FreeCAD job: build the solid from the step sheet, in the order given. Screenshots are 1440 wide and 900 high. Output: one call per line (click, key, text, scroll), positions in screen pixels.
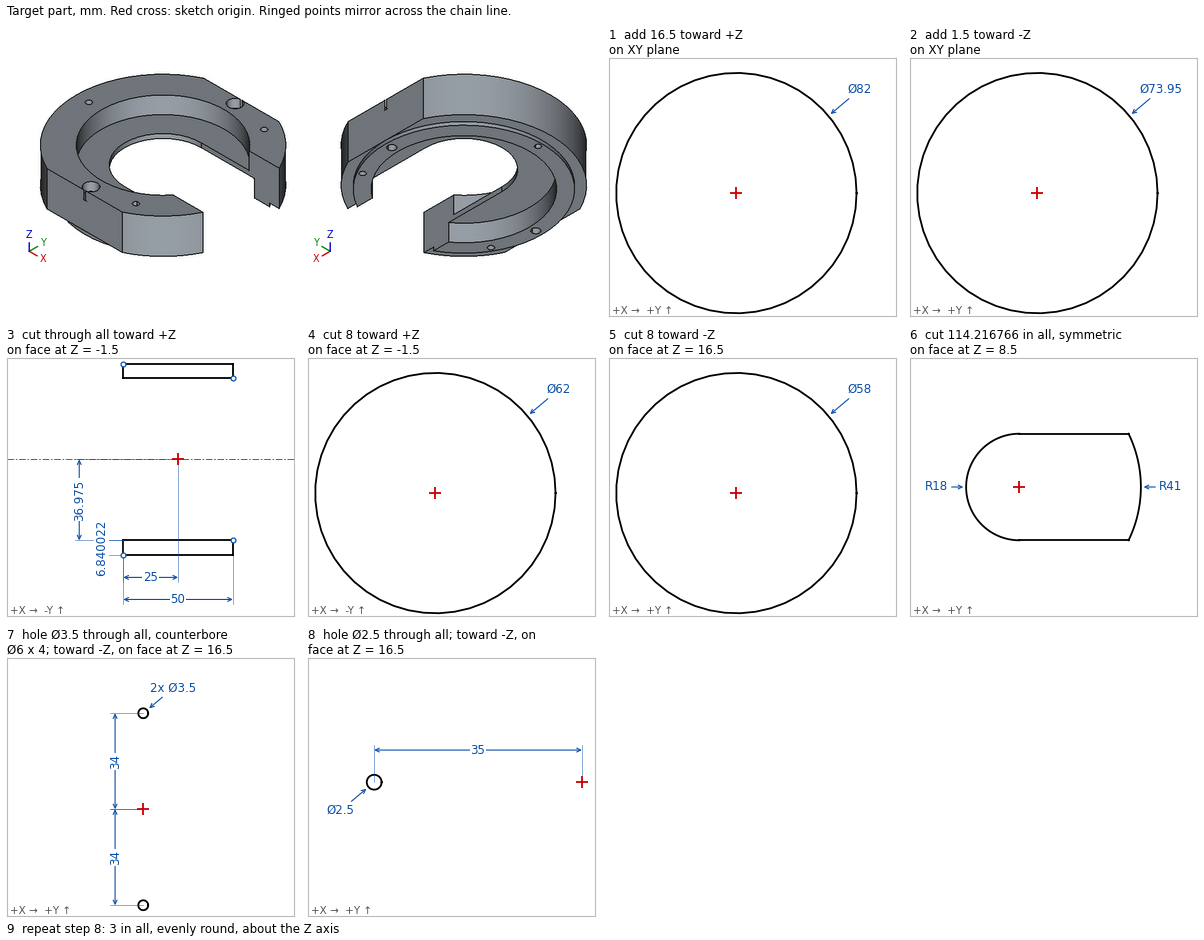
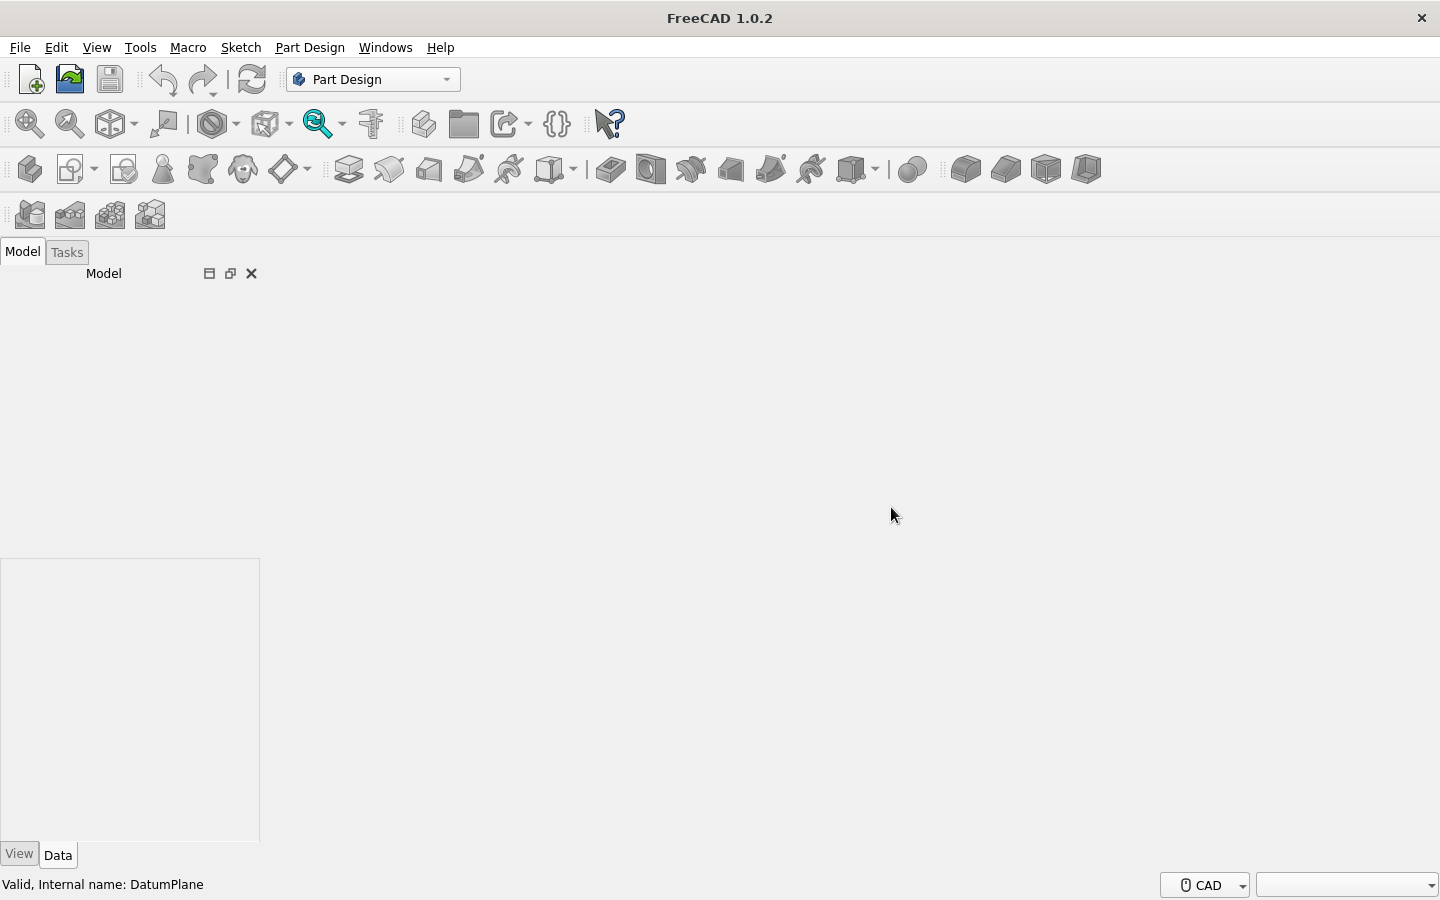
key(ctrl+n)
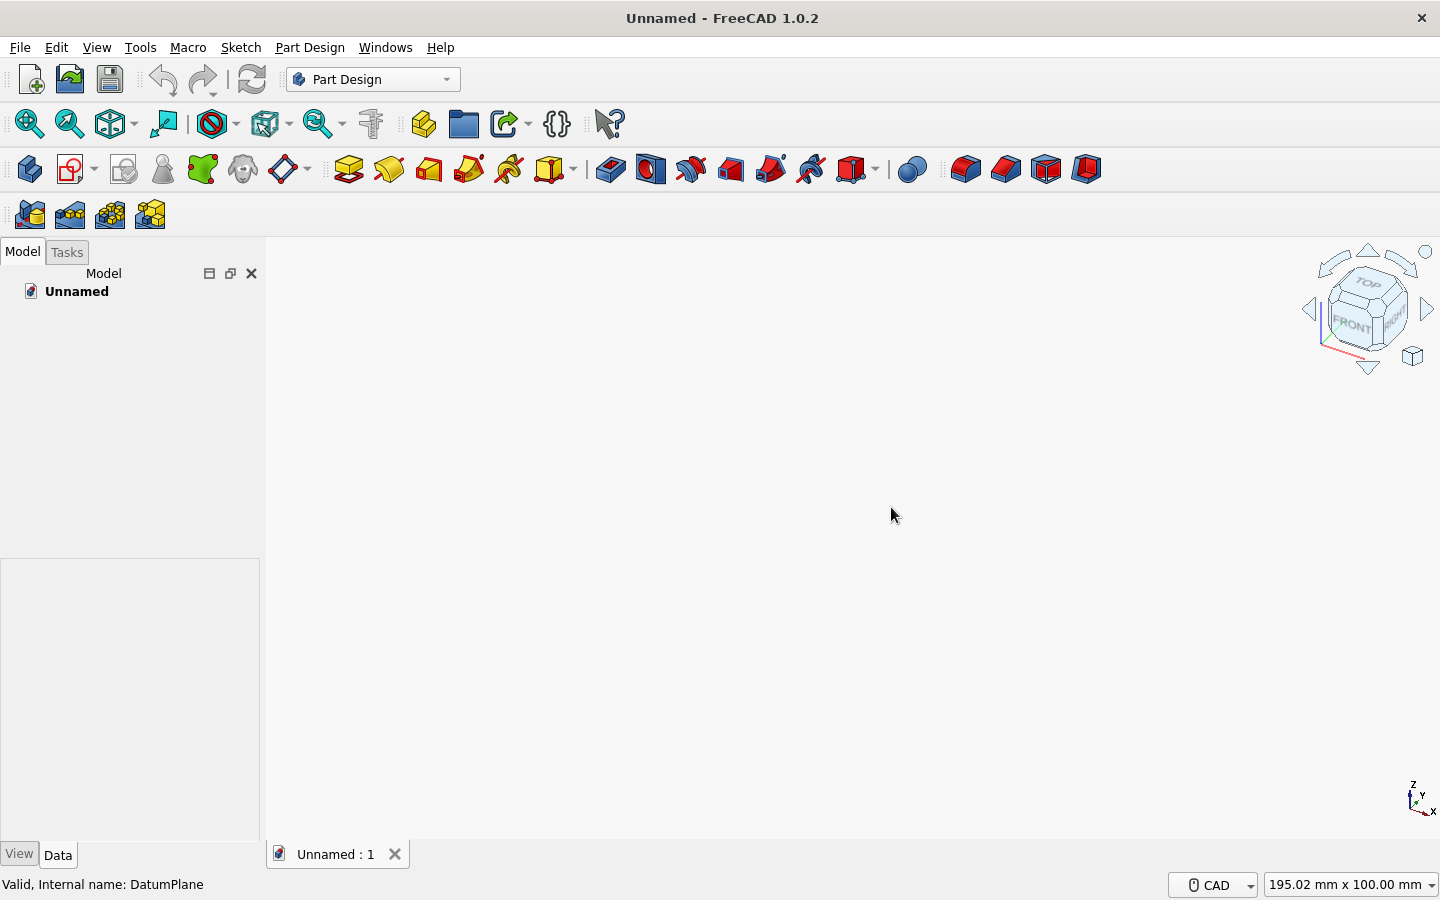
click(70, 170)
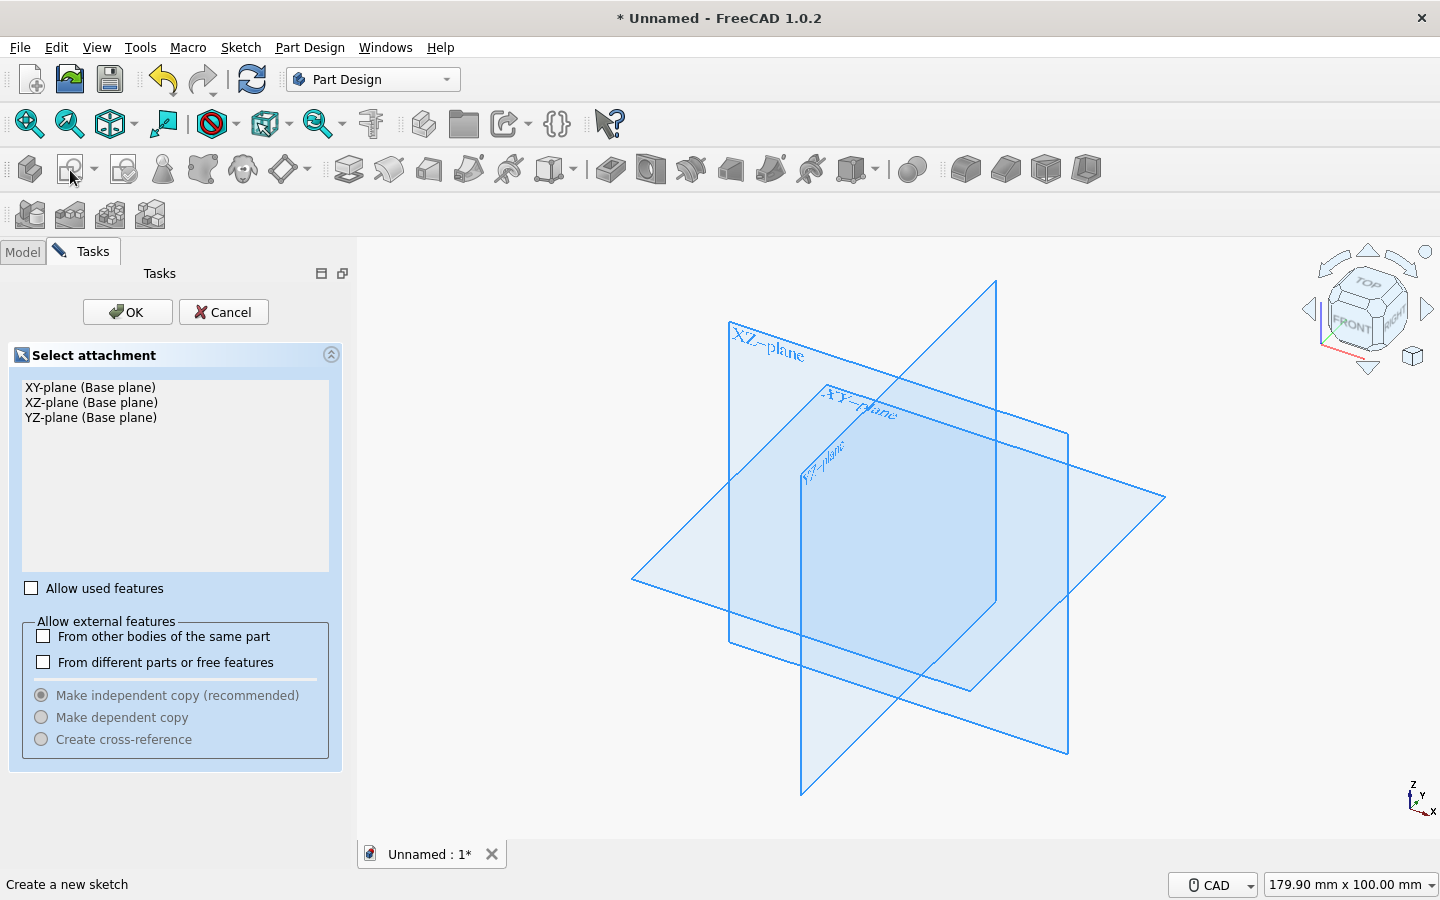
click(82, 388)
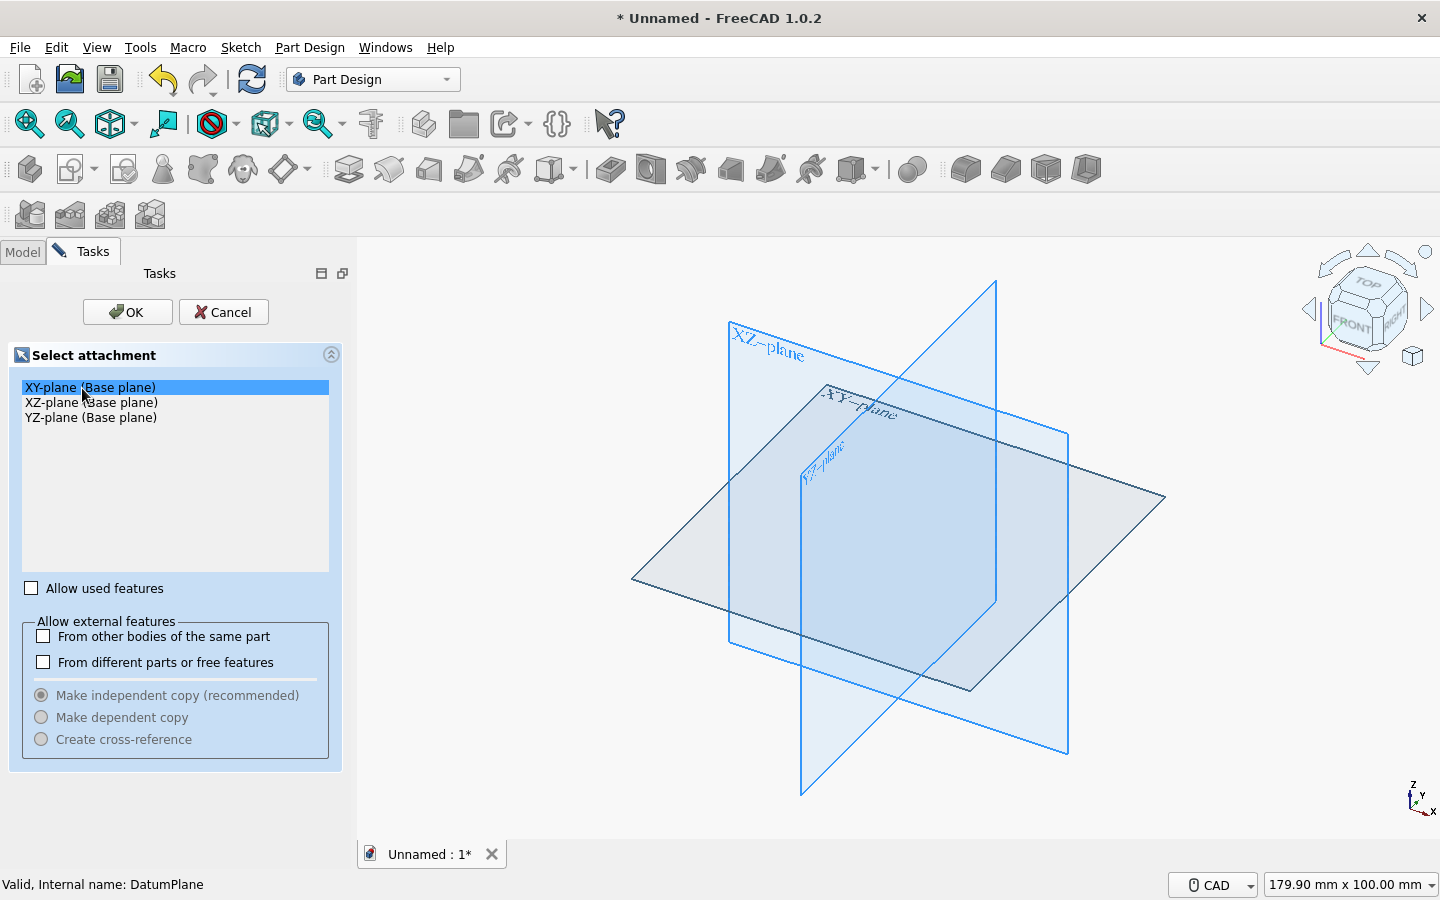
click(128, 312)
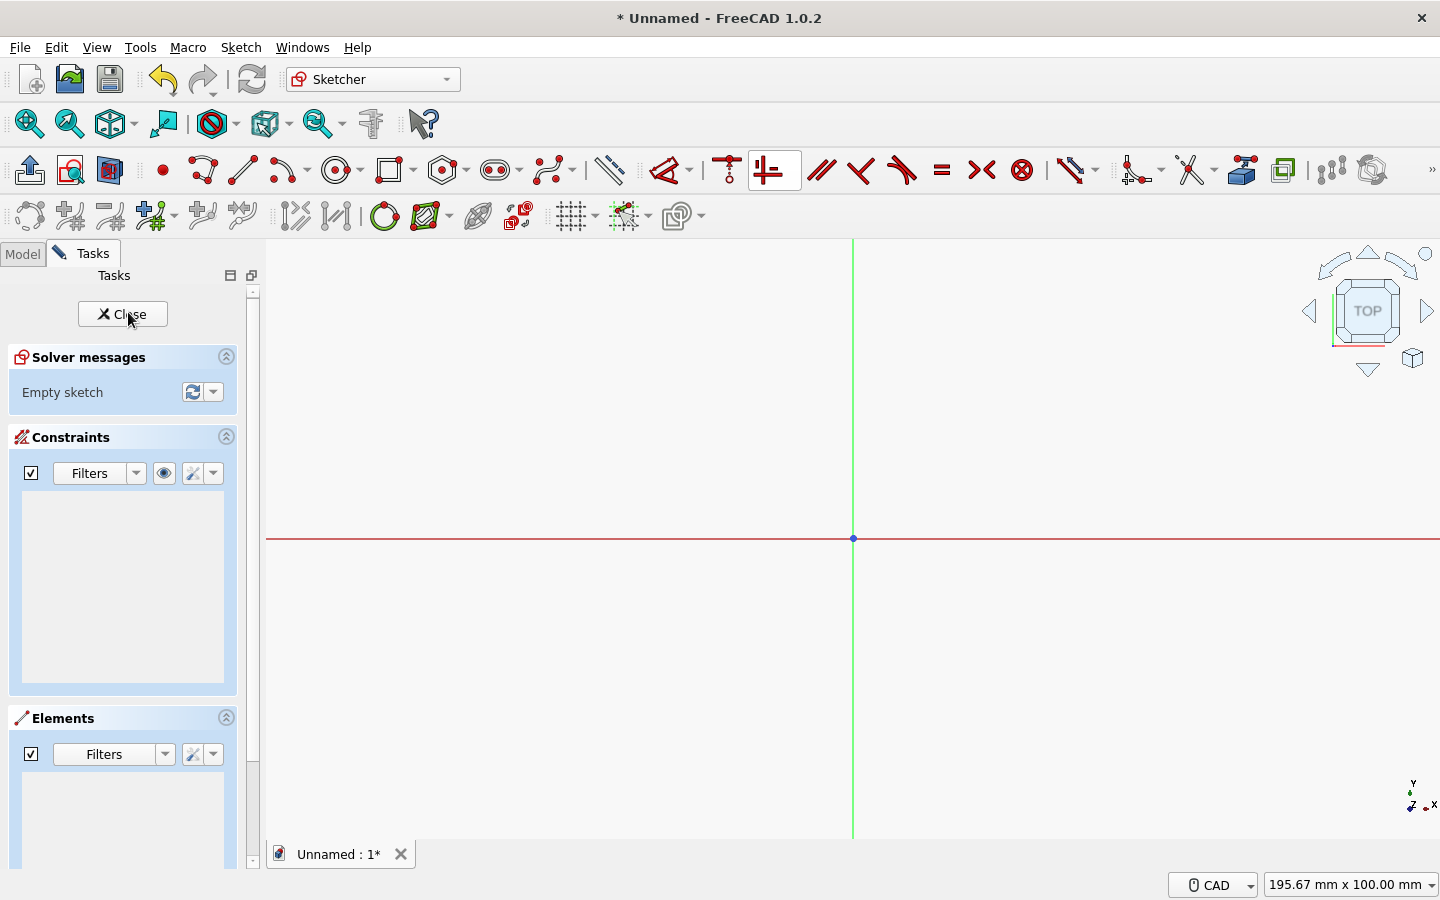
key(g)
key(c)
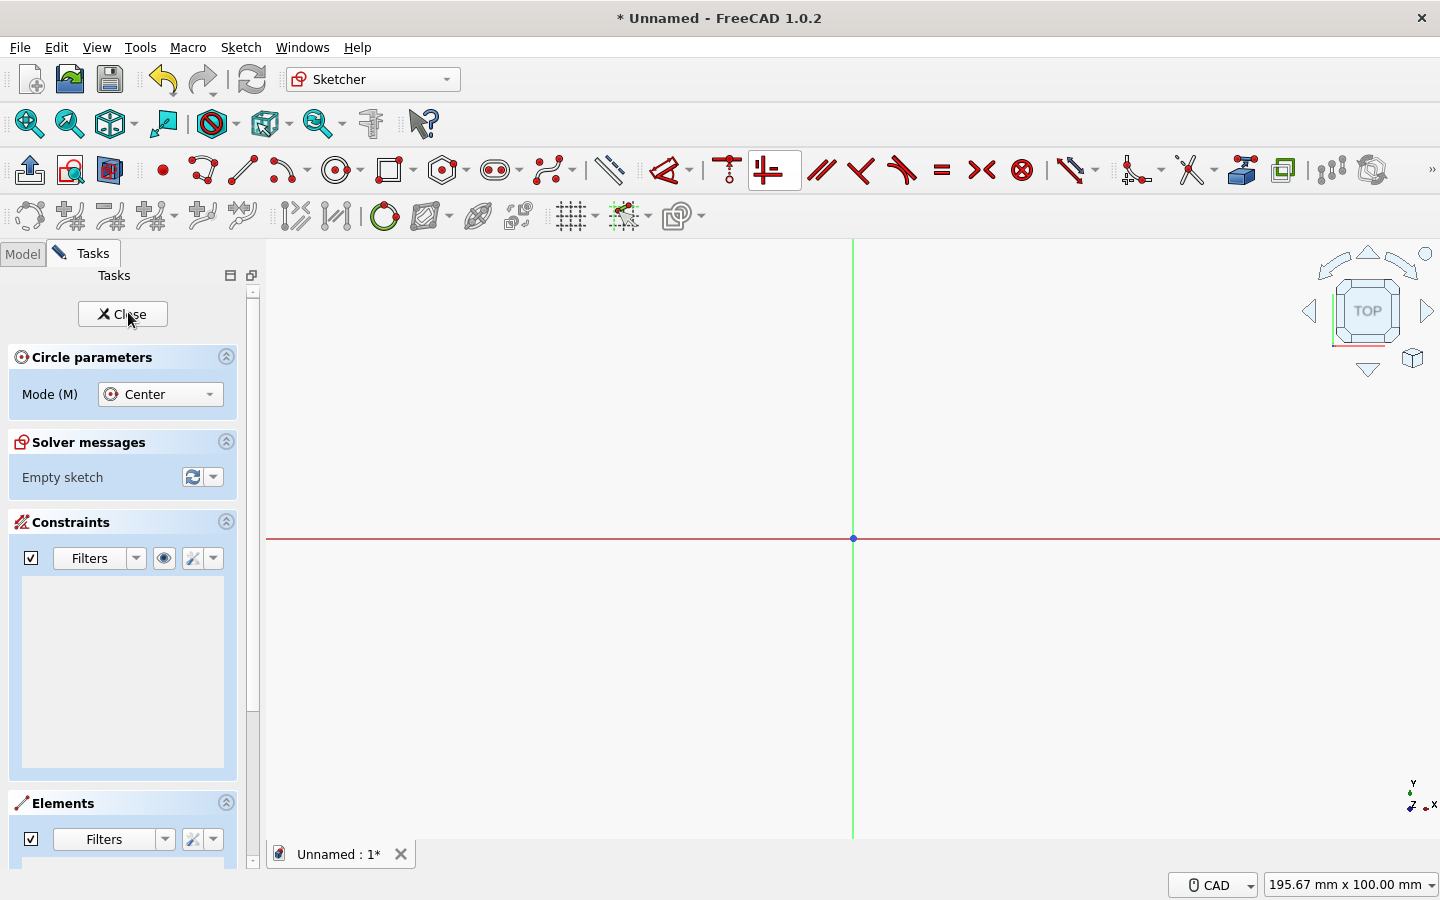
click(853, 539)
click(1027, 365)
key(Escape)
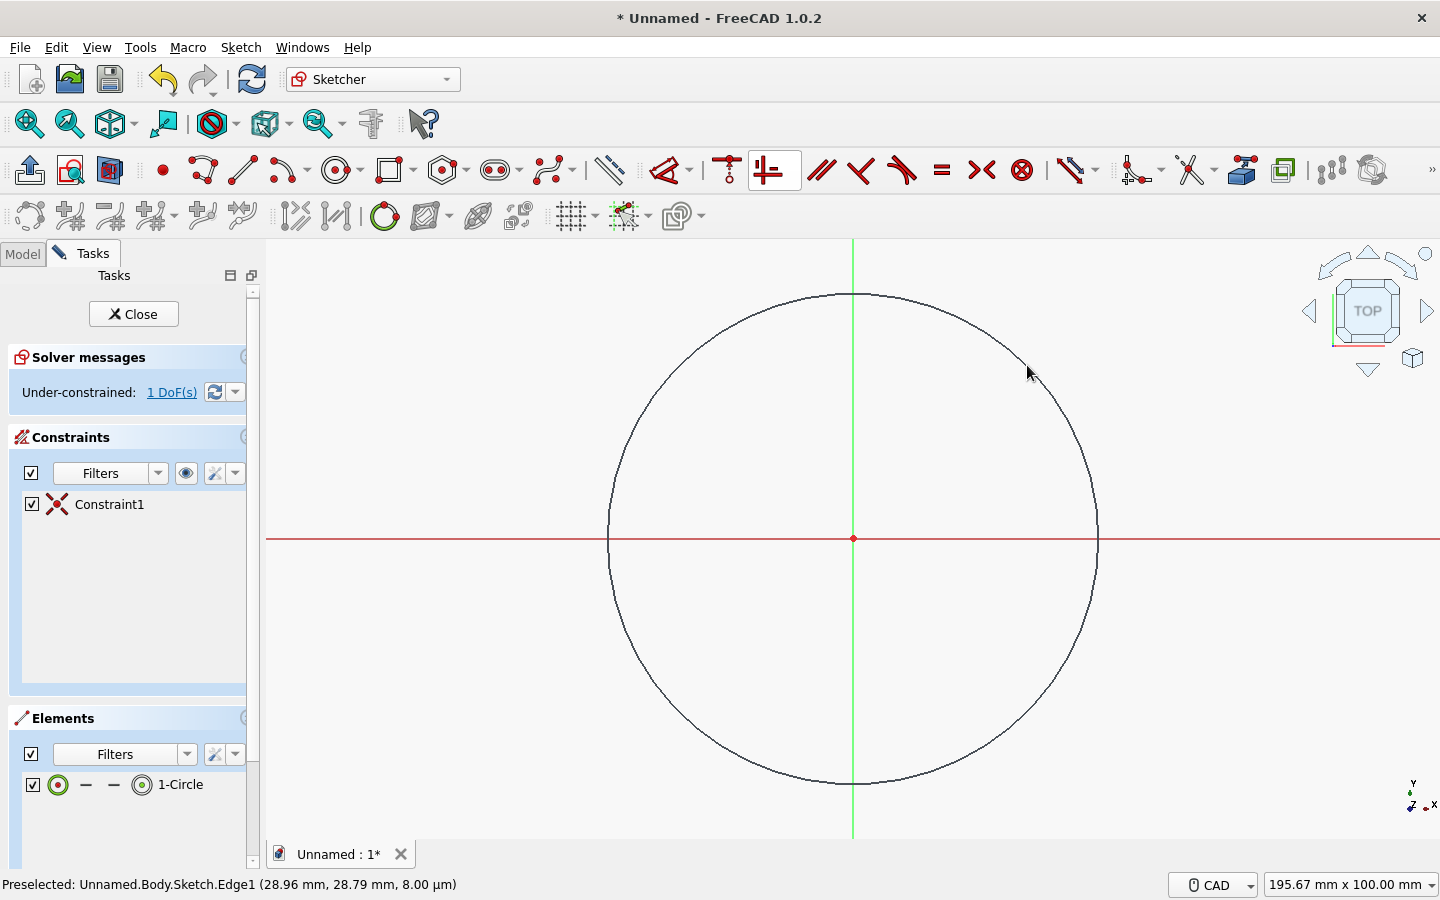
key(d)